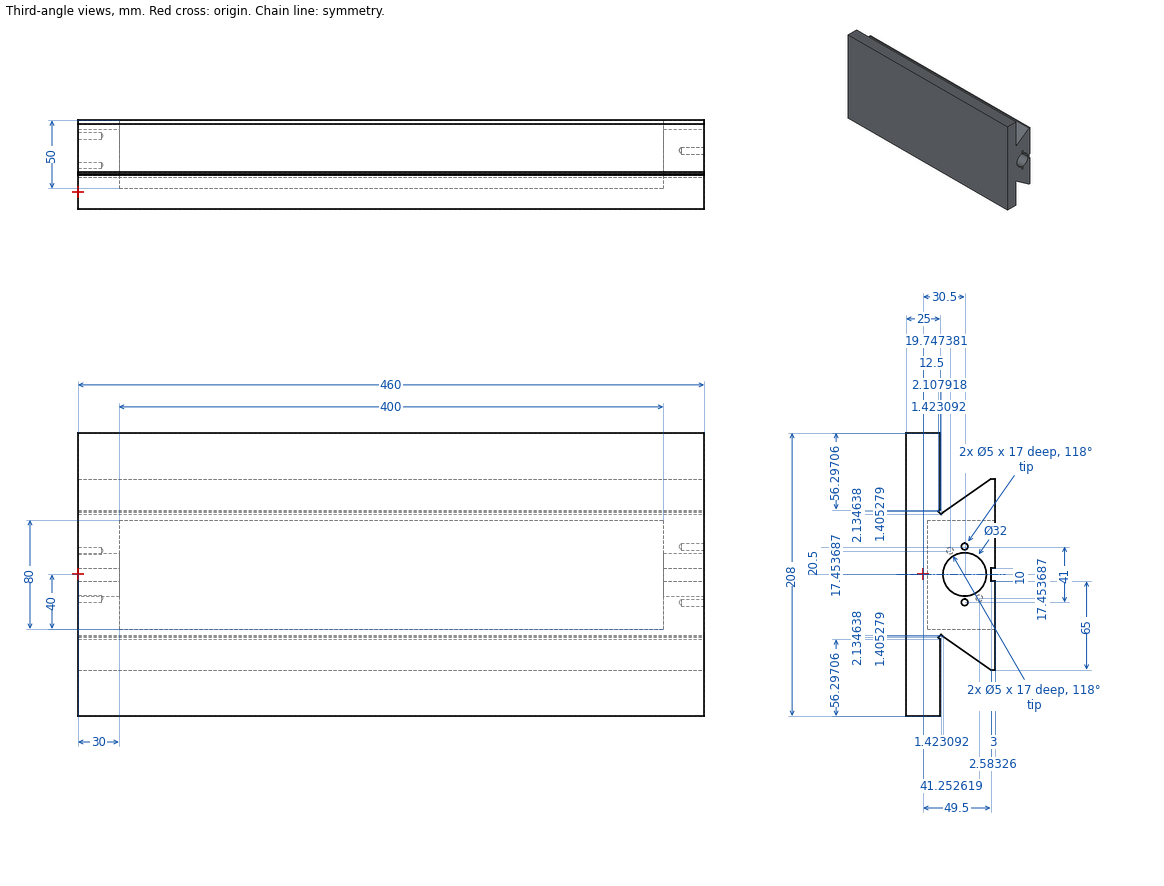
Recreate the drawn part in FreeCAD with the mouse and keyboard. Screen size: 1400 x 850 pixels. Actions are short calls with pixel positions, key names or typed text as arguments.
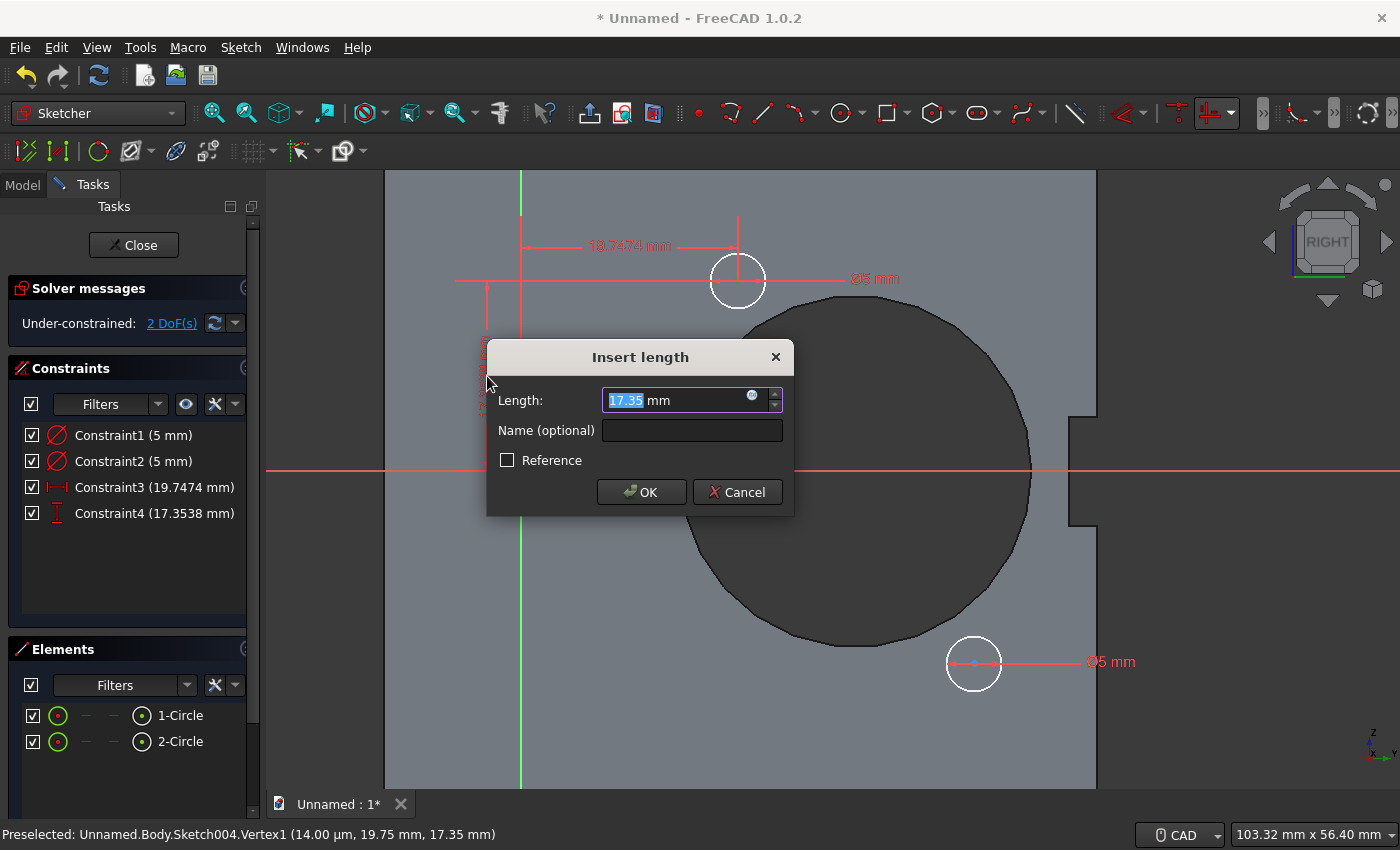
text(17.453687)
key(Return)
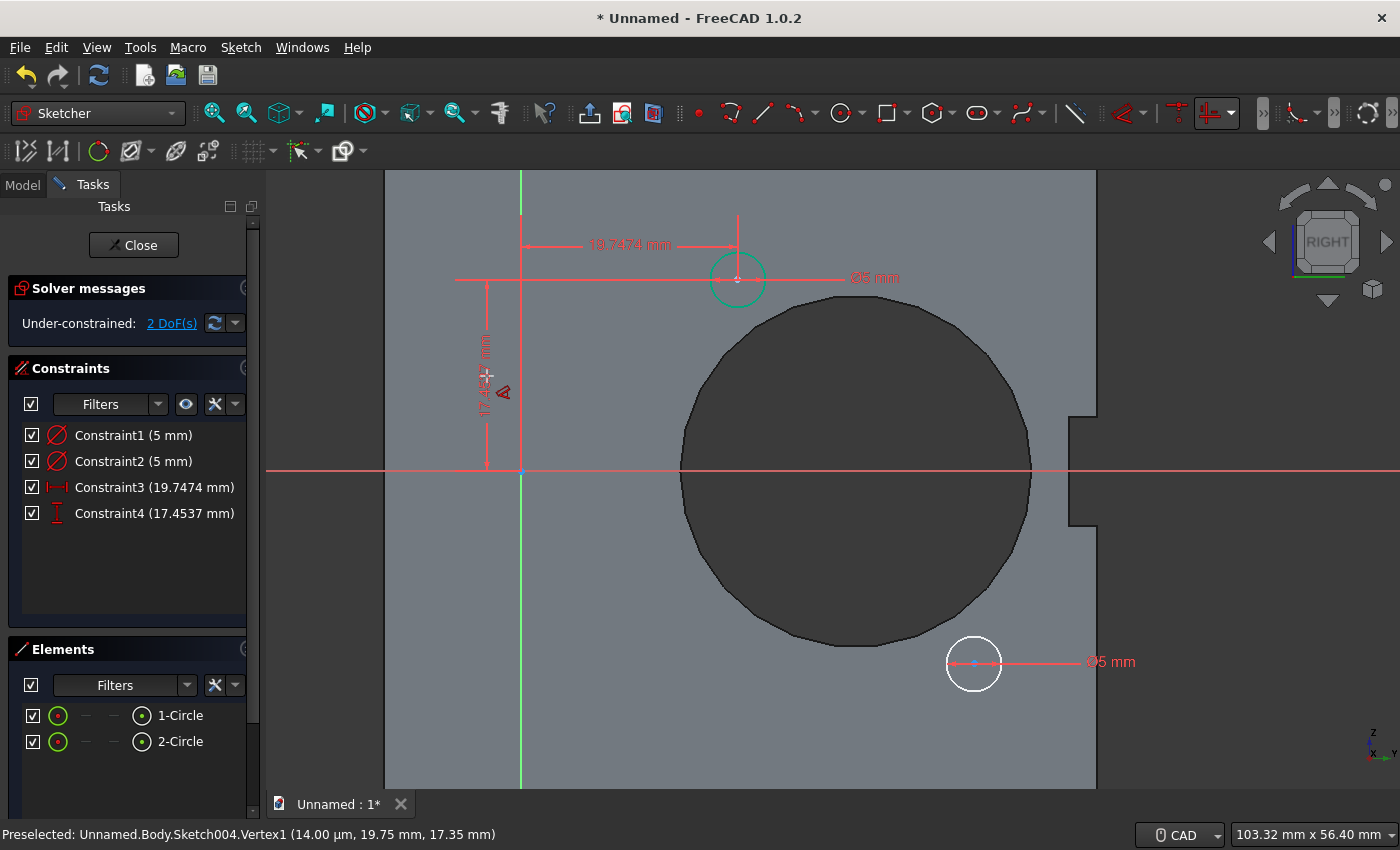
click(974, 664)
click(748, 698)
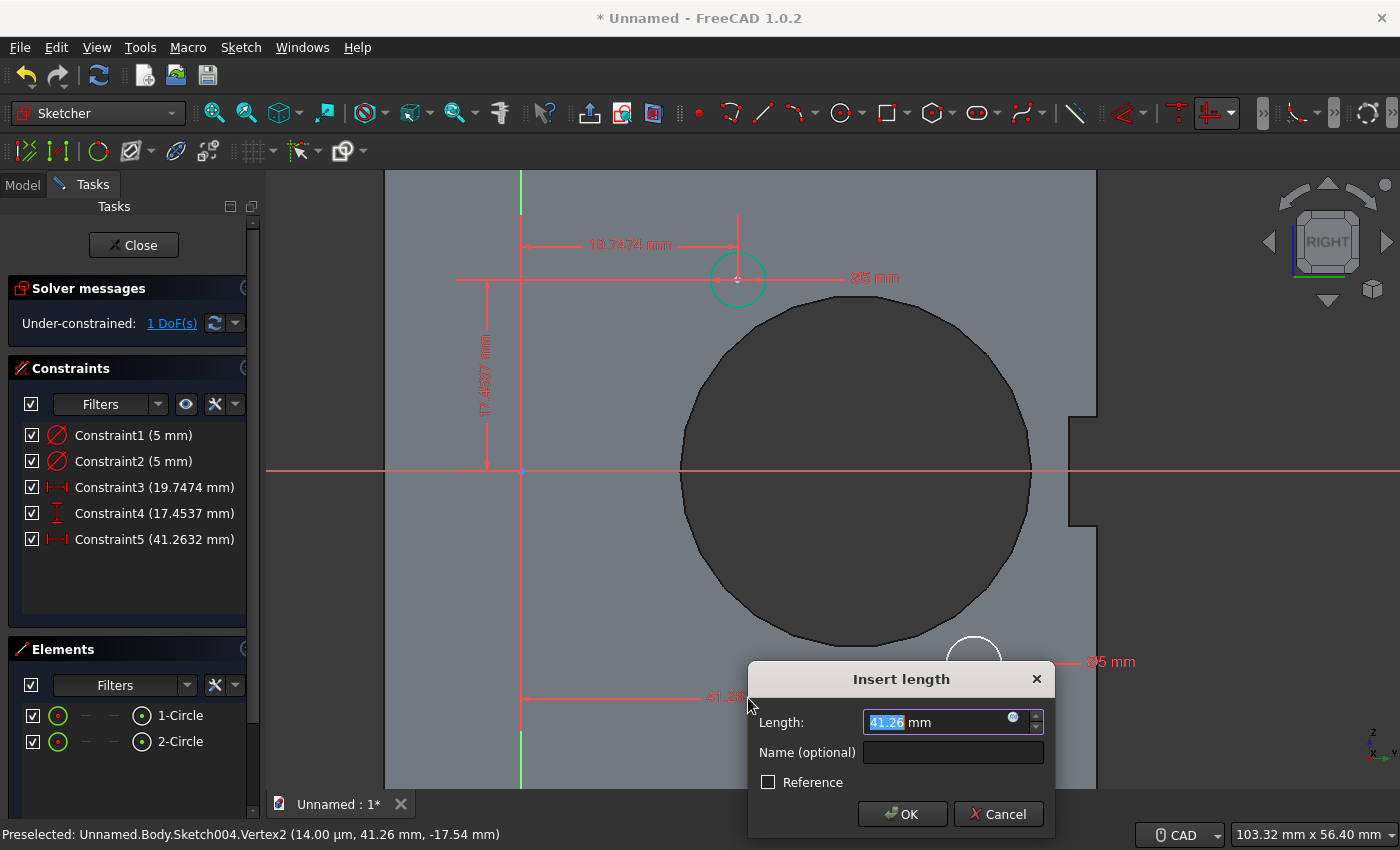
text(41.252619)
key(Return)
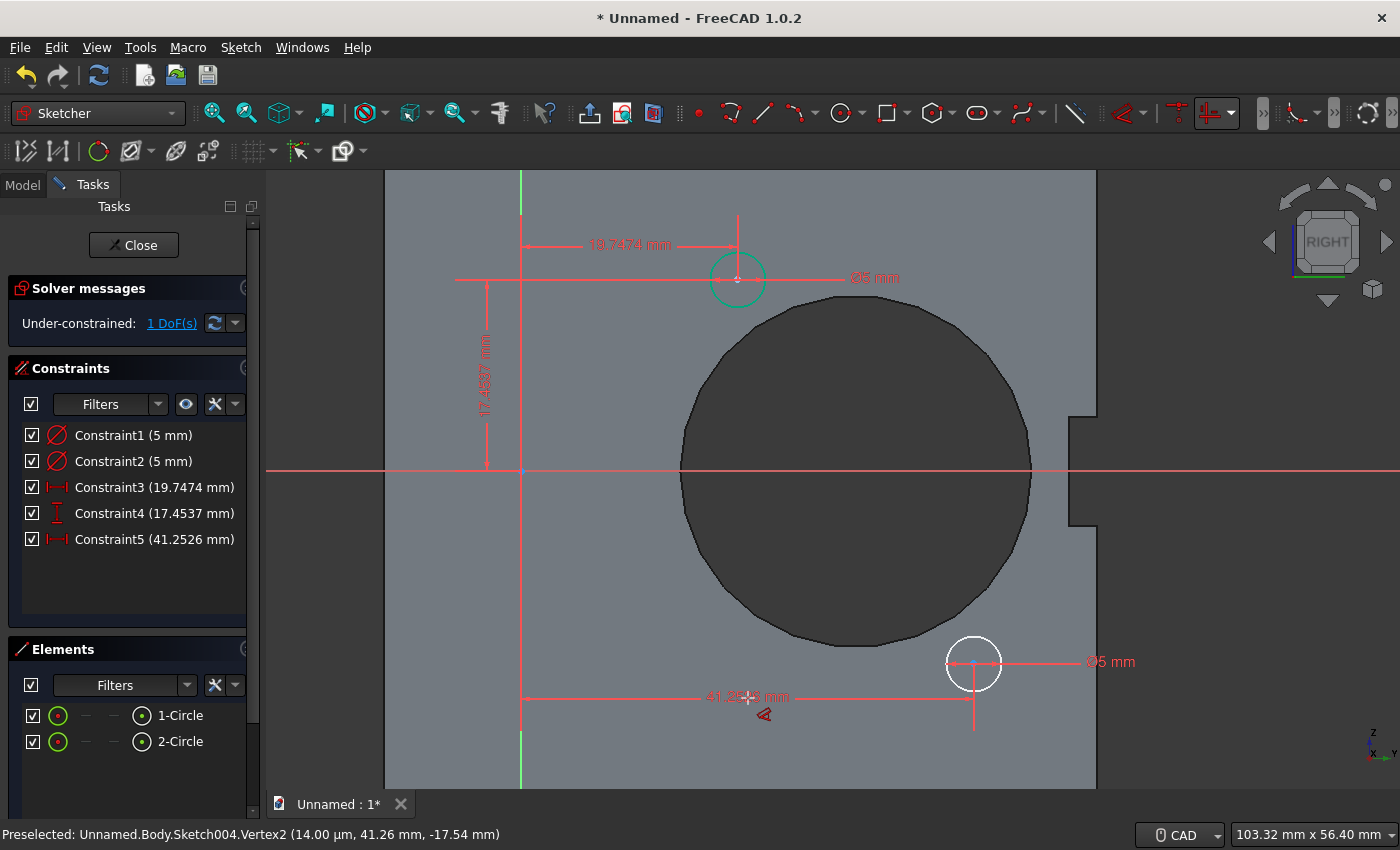
click(974, 664)
click(487, 568)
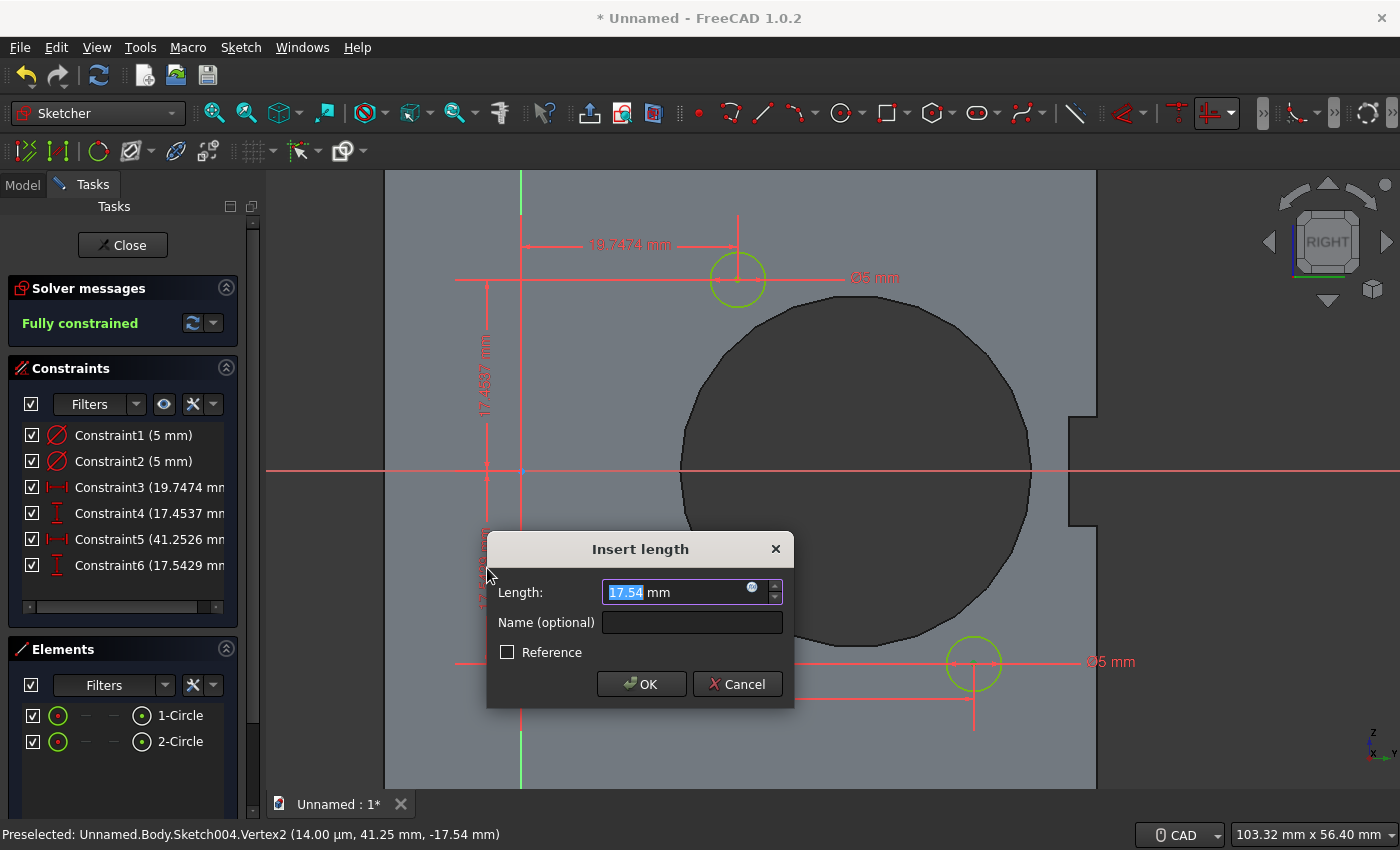
text(17.453687)
key(Return)
key(Escape)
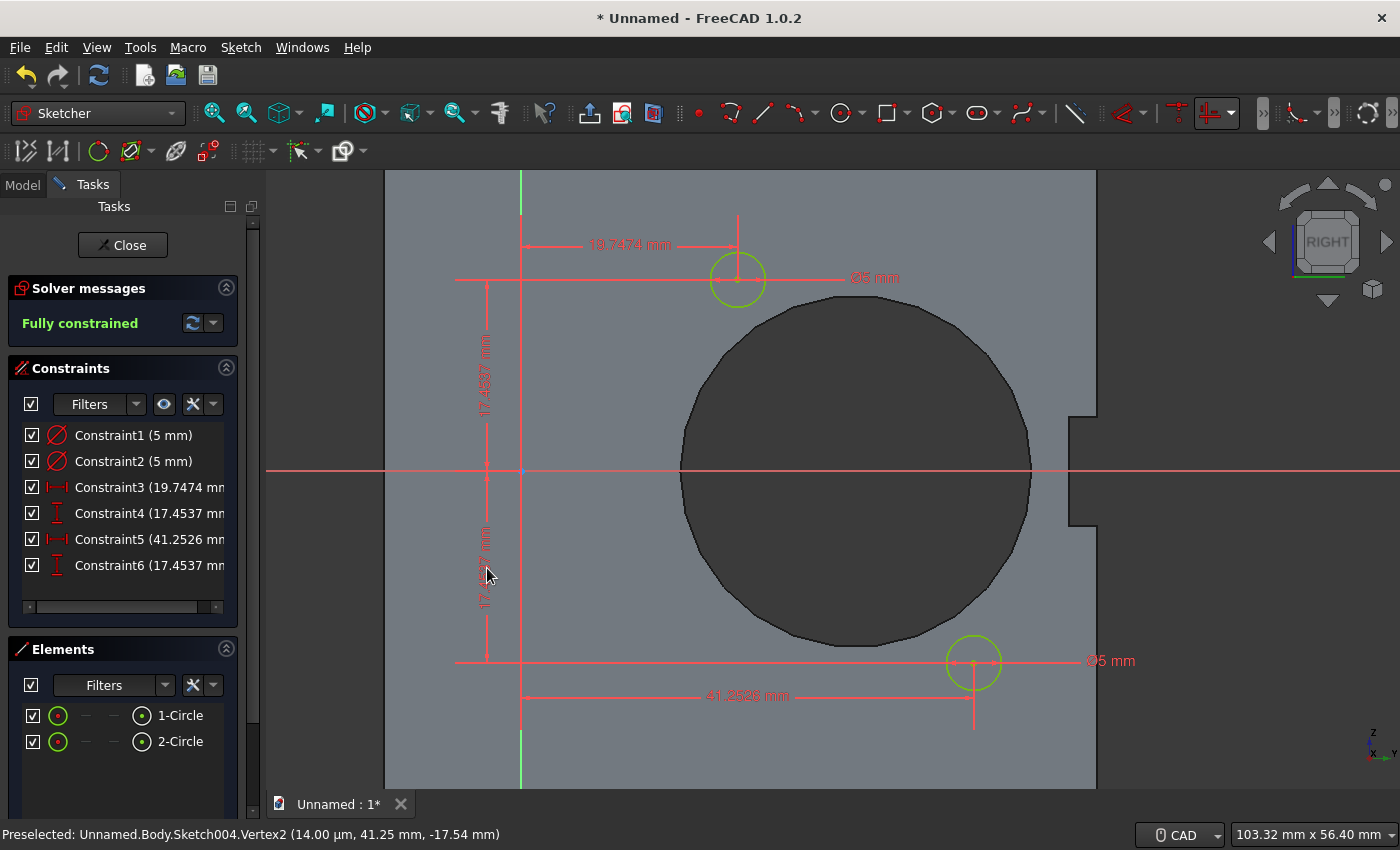
click(123, 245)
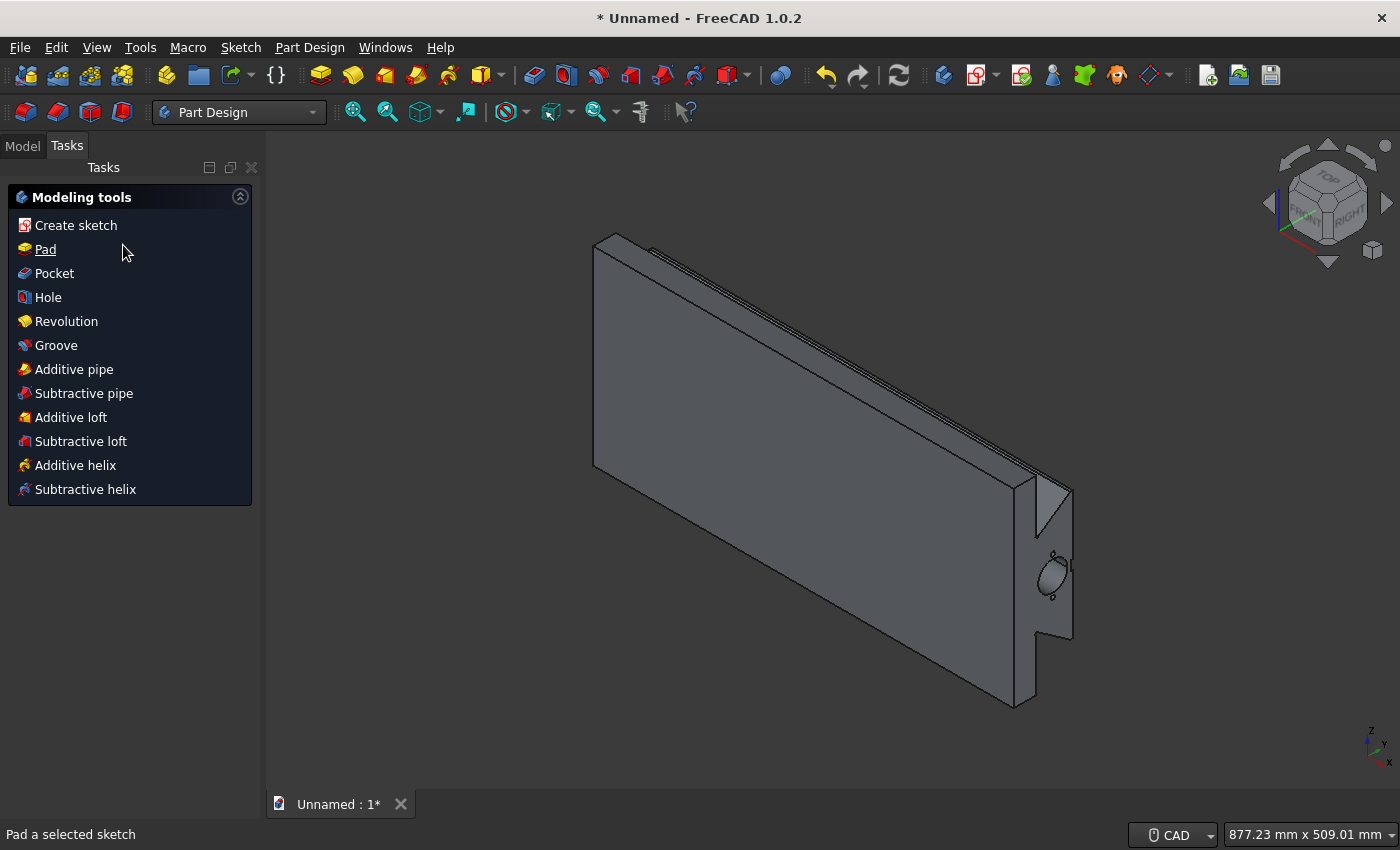
click(568, 76)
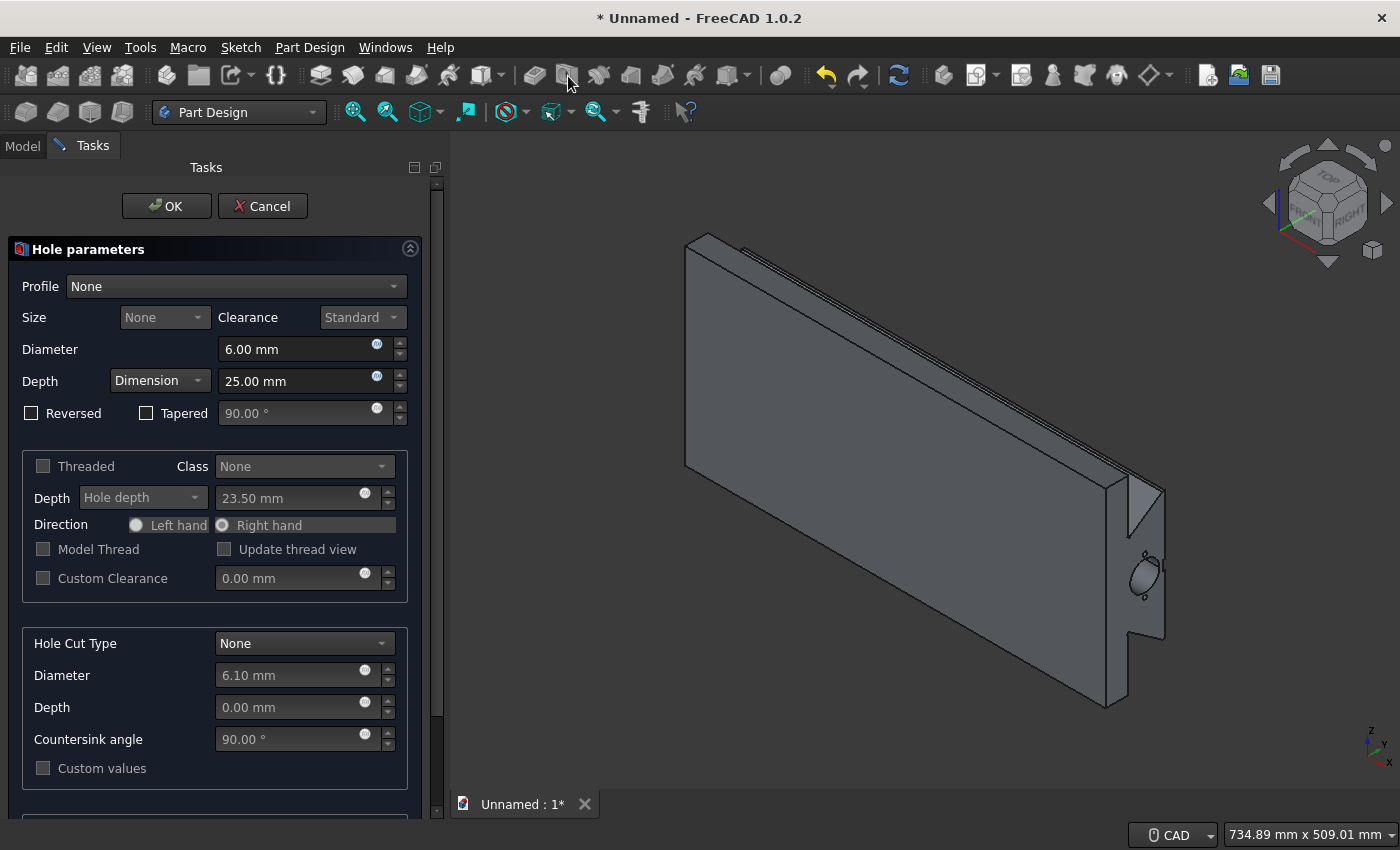
triple_click(305, 349)